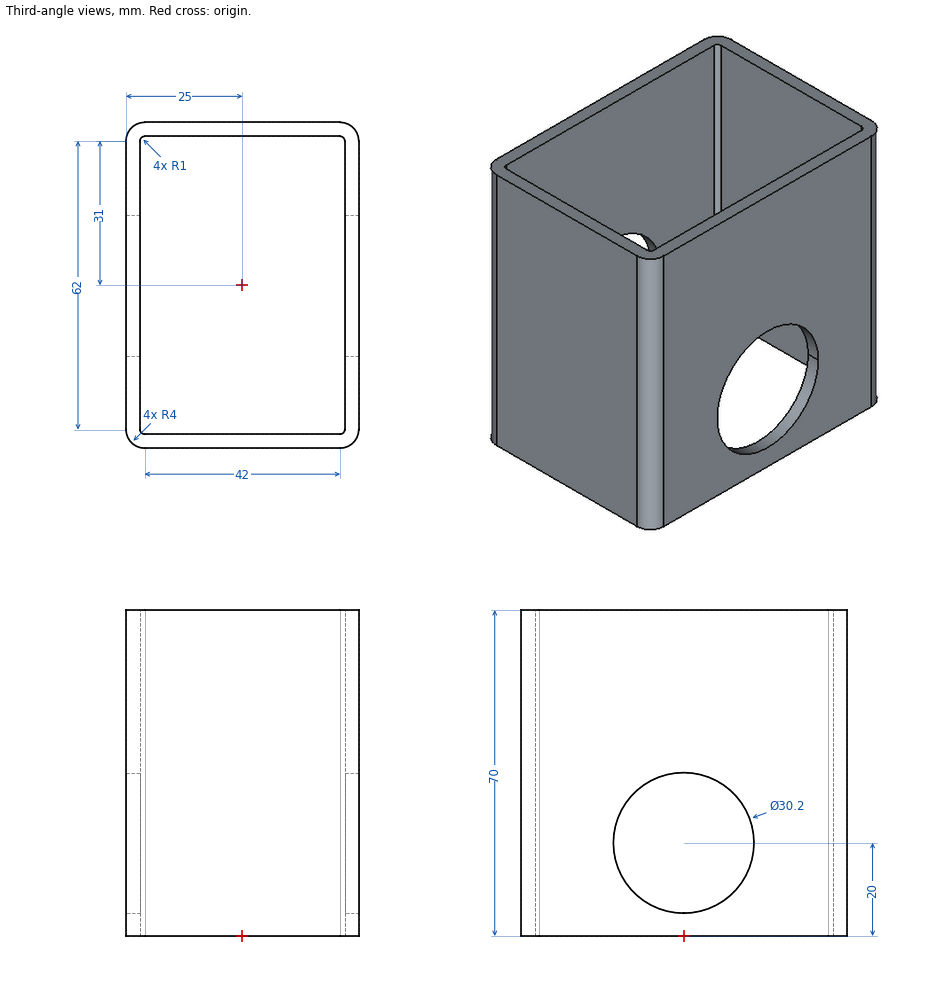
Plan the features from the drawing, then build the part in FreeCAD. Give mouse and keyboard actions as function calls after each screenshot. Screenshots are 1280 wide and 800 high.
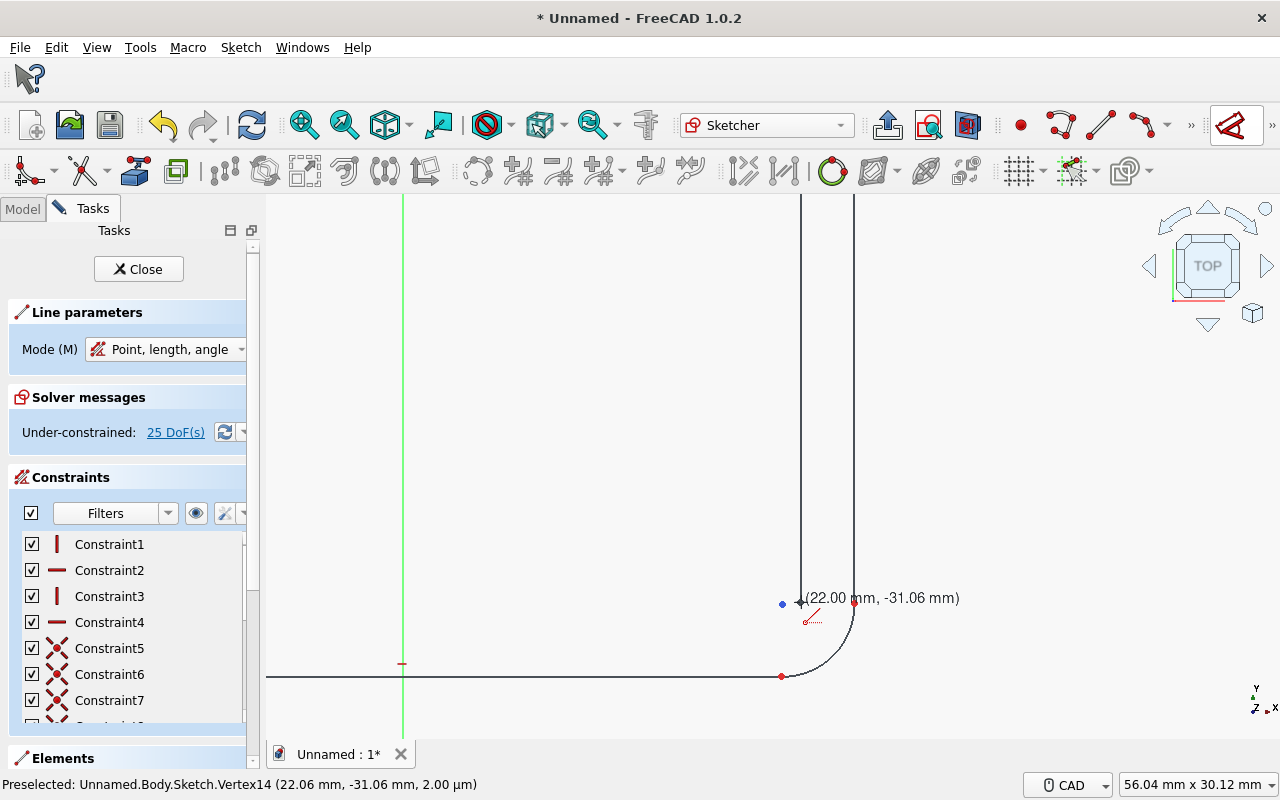
click(783, 620)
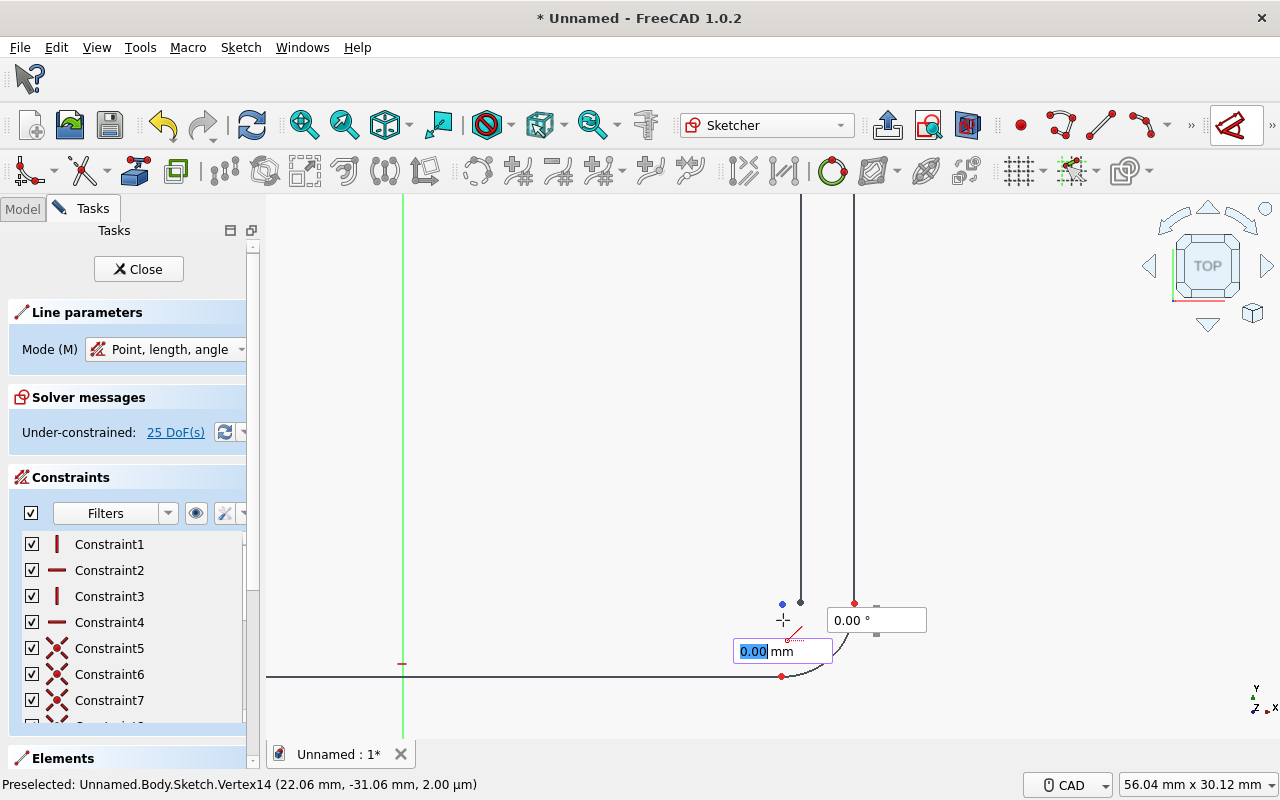
scroll(803, 606, down, 7)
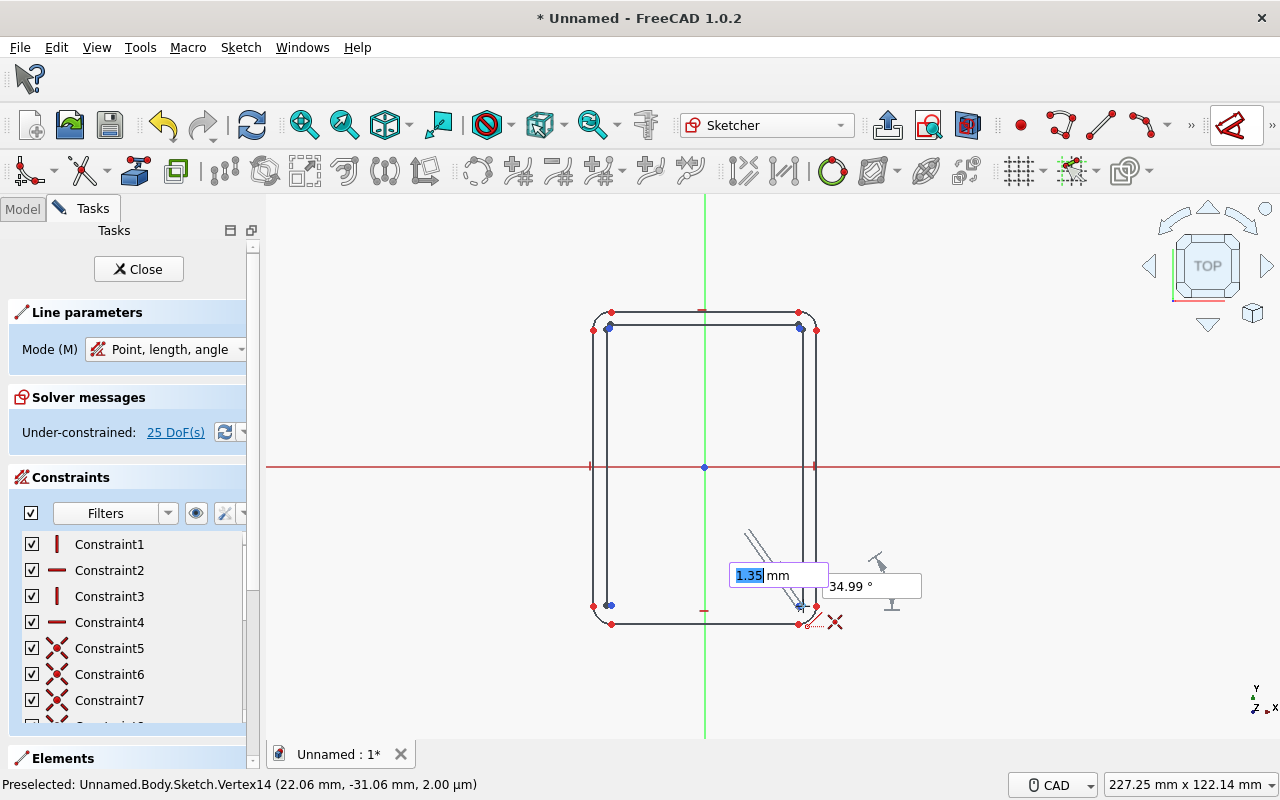
scroll(611, 610, up, 7)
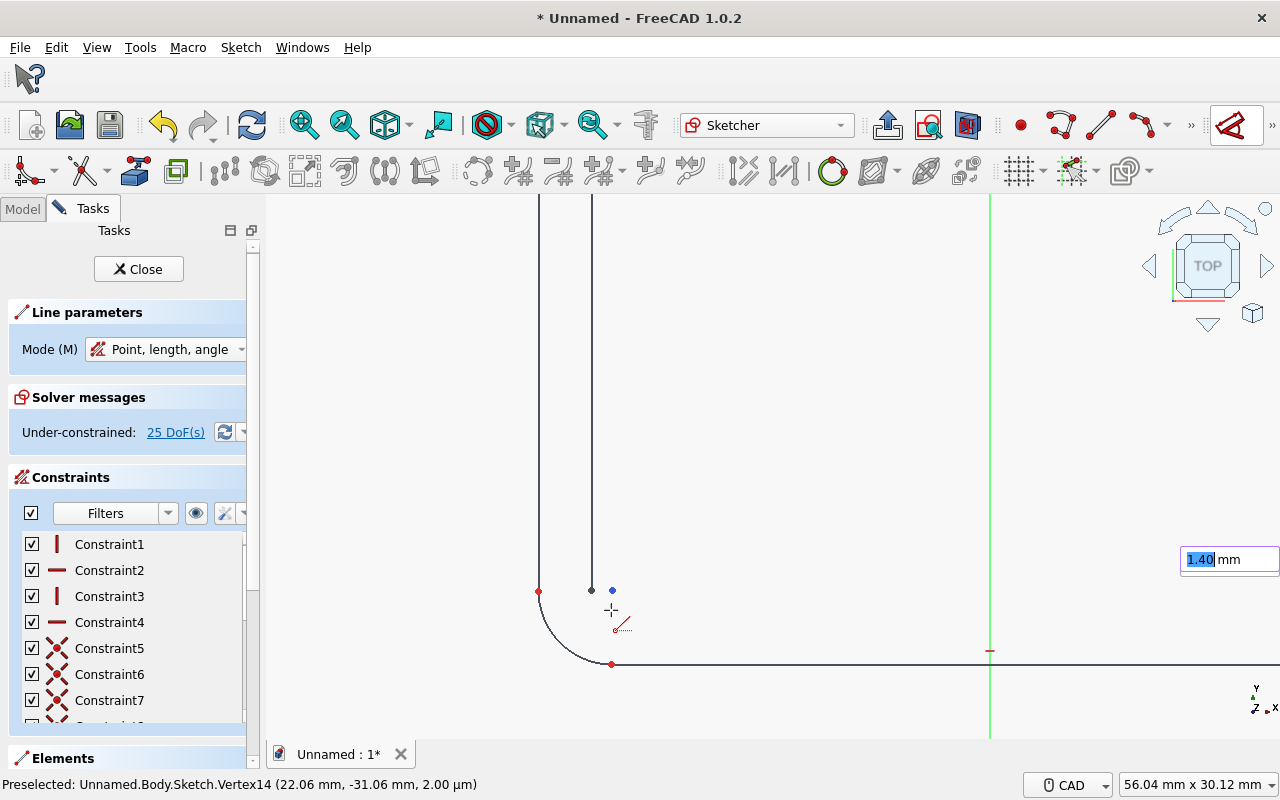
click(610, 608)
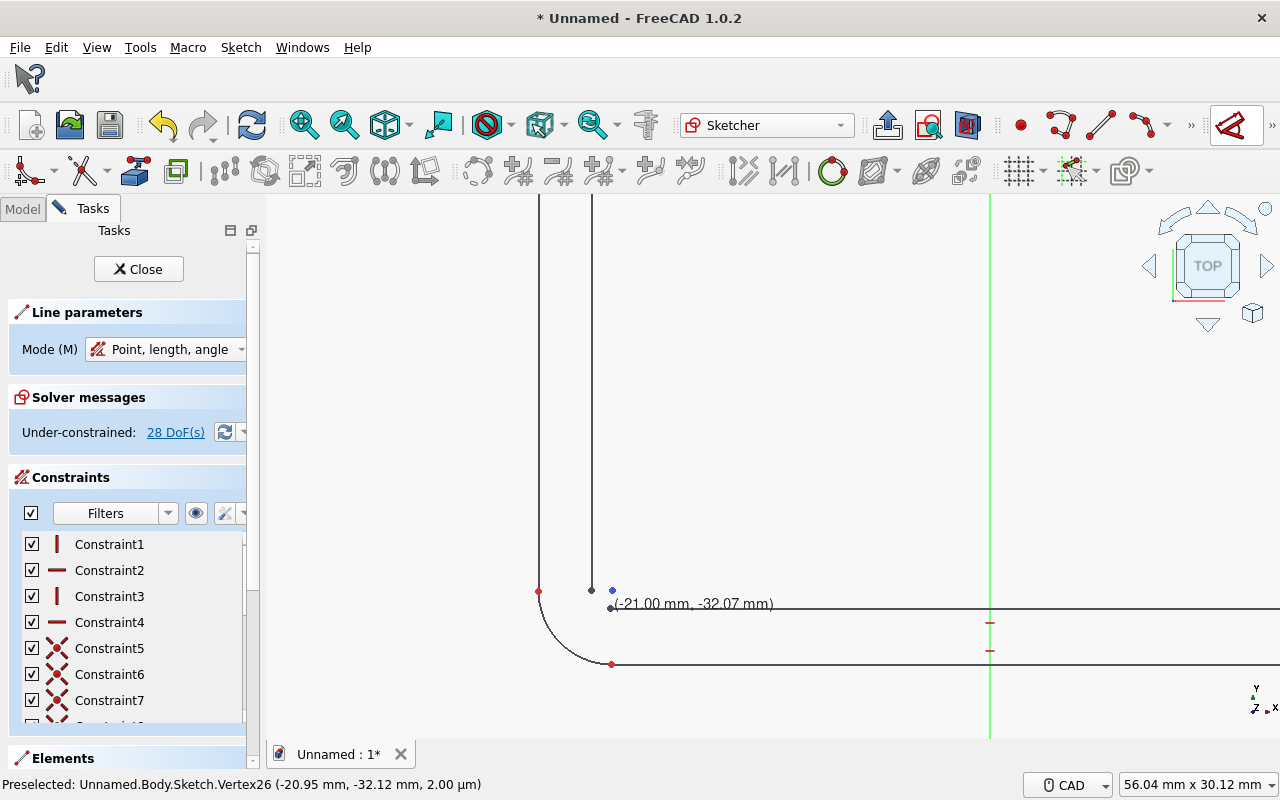
key(g)
key(3)
key(a)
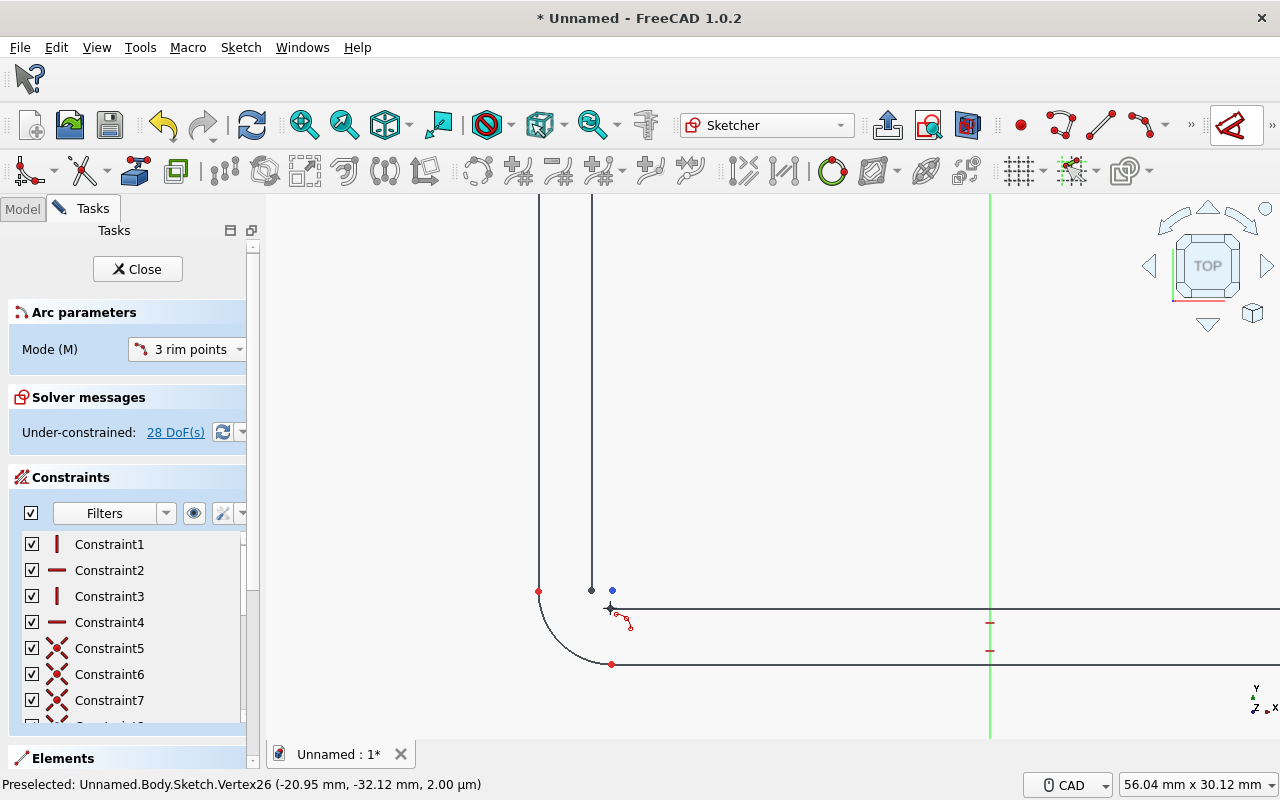
scroll(611, 610, down, 7)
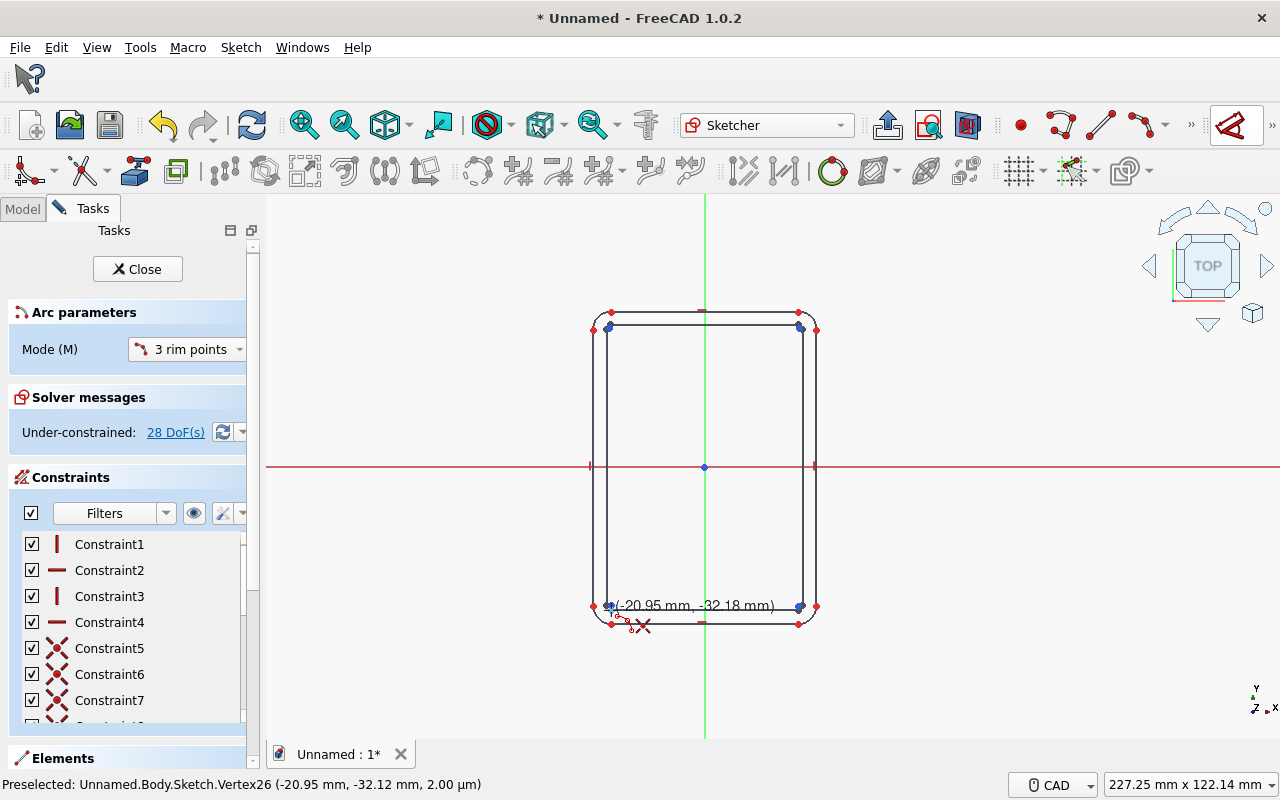
scroll(607, 329, up, 7)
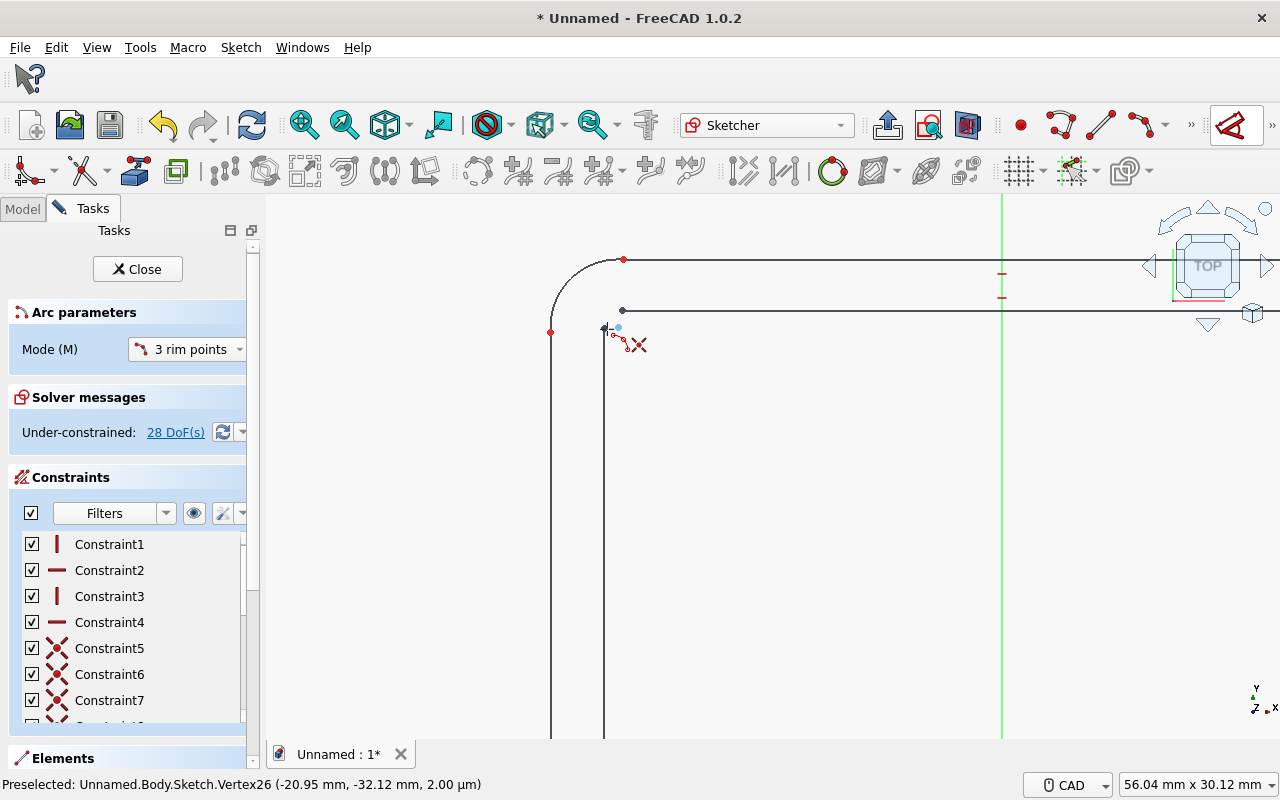
click(604, 329)
click(622, 311)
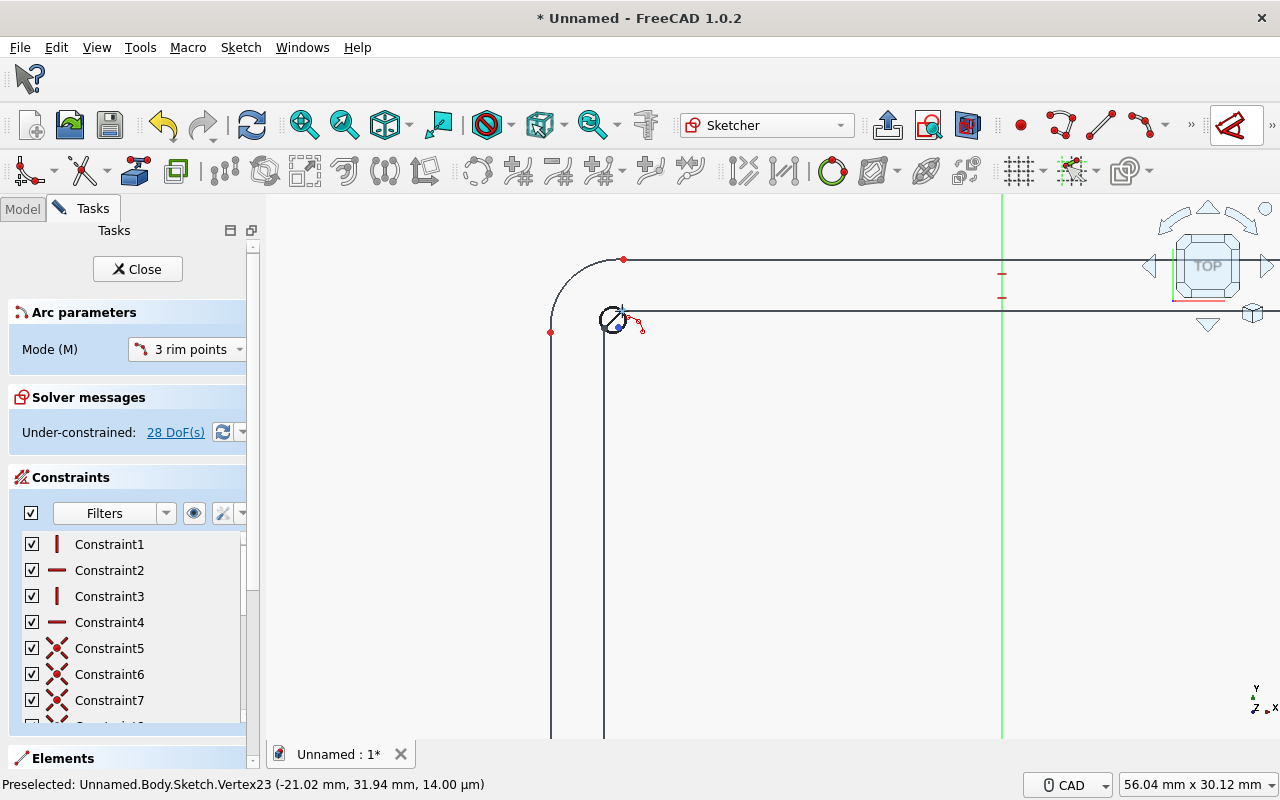
scroll(610, 315, up, 6)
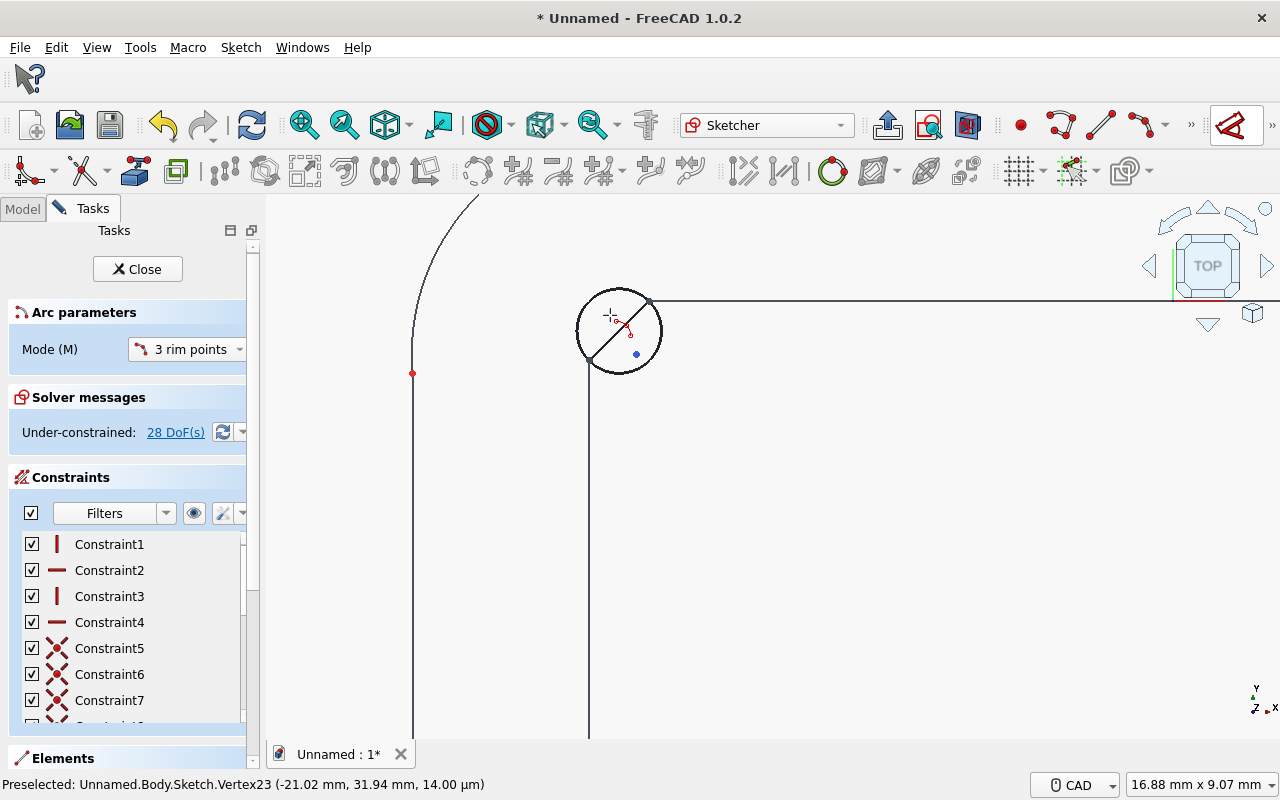
click(608, 315)